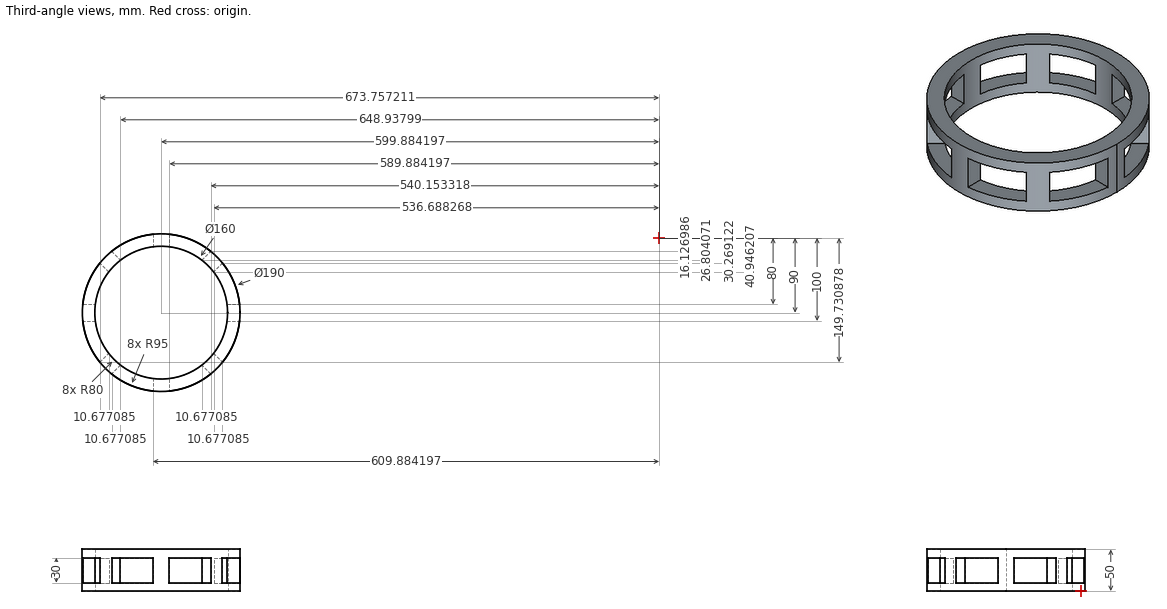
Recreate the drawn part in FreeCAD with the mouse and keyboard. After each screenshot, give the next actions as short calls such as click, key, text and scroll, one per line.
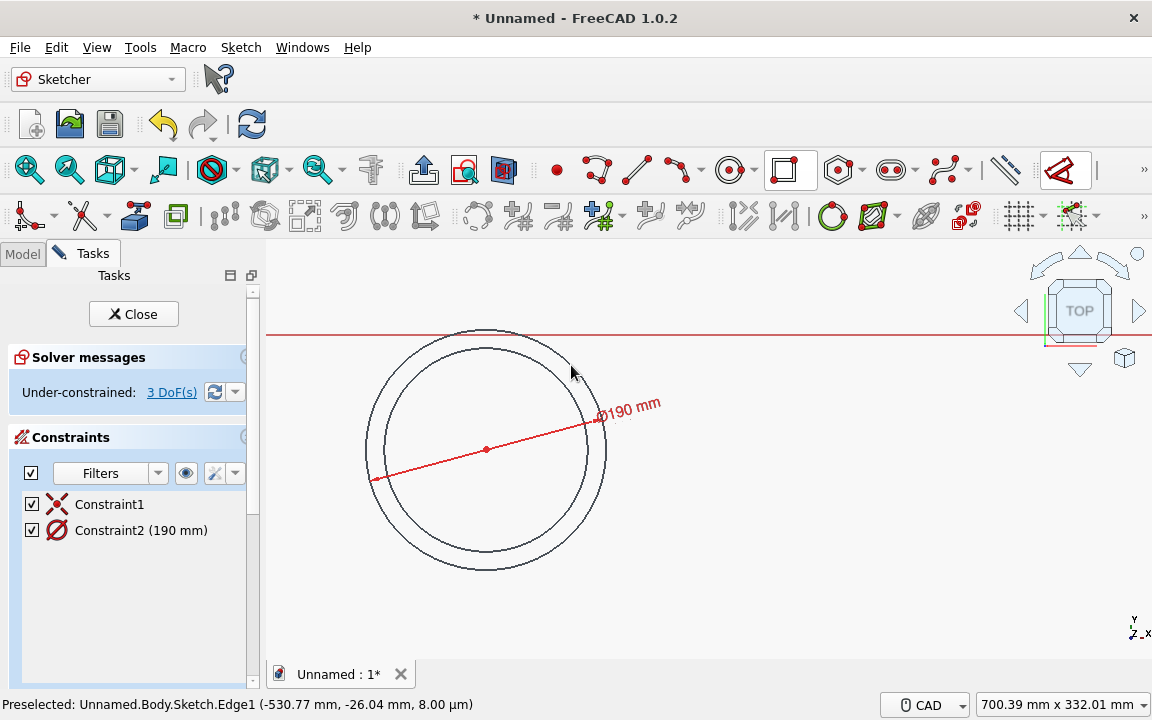
click(558, 378)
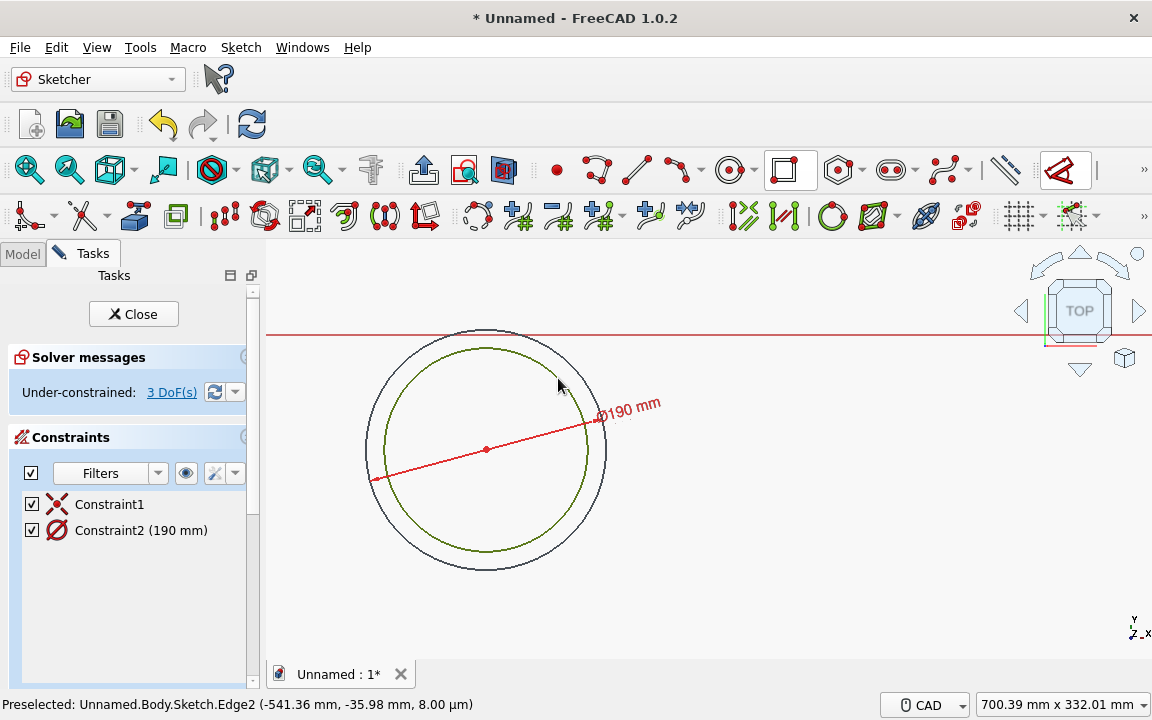
key(k)
key(o)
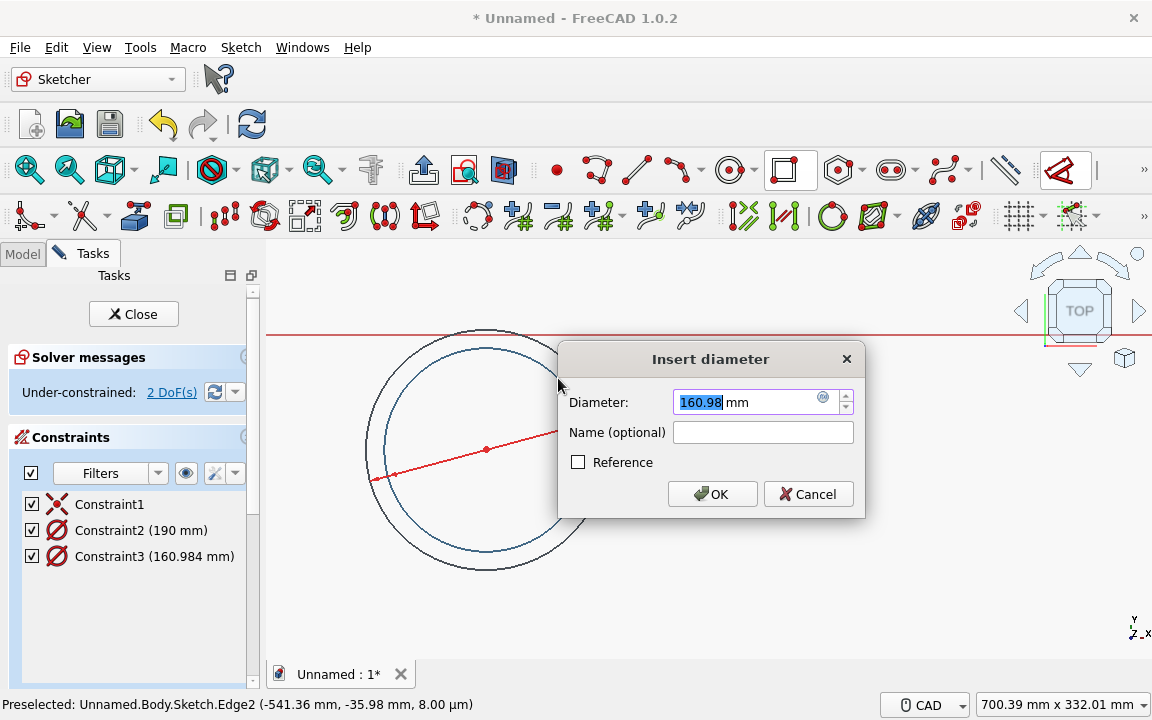
text(160)
key(Return)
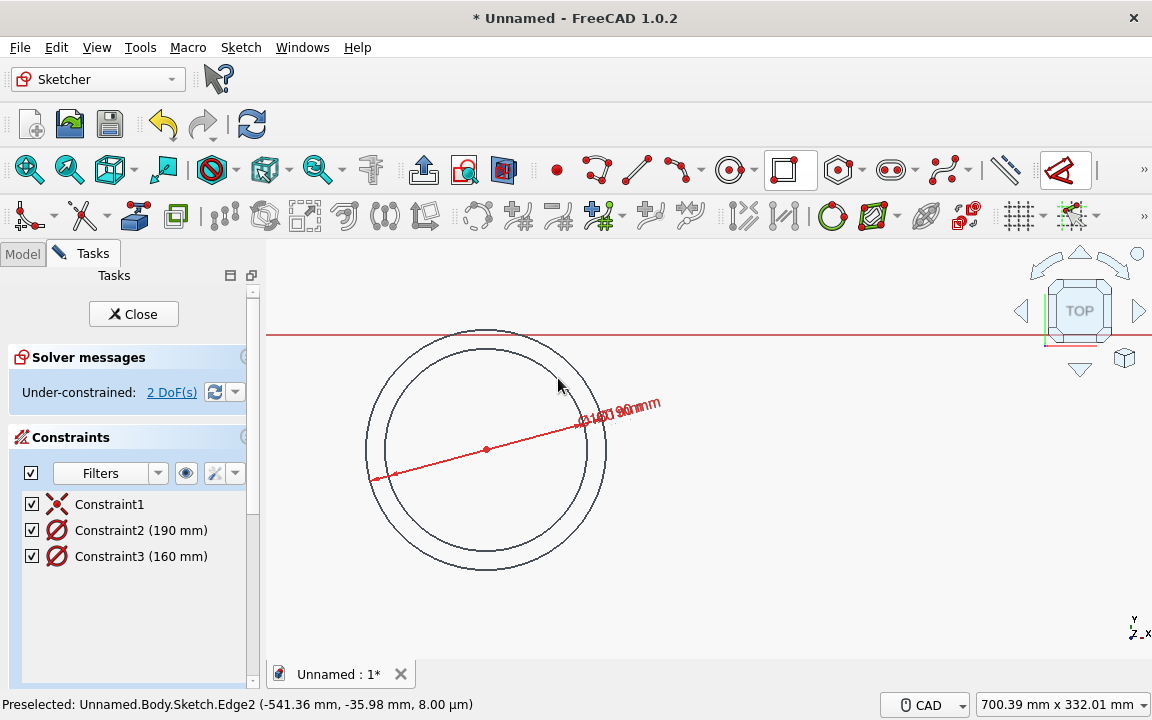
click(486, 450)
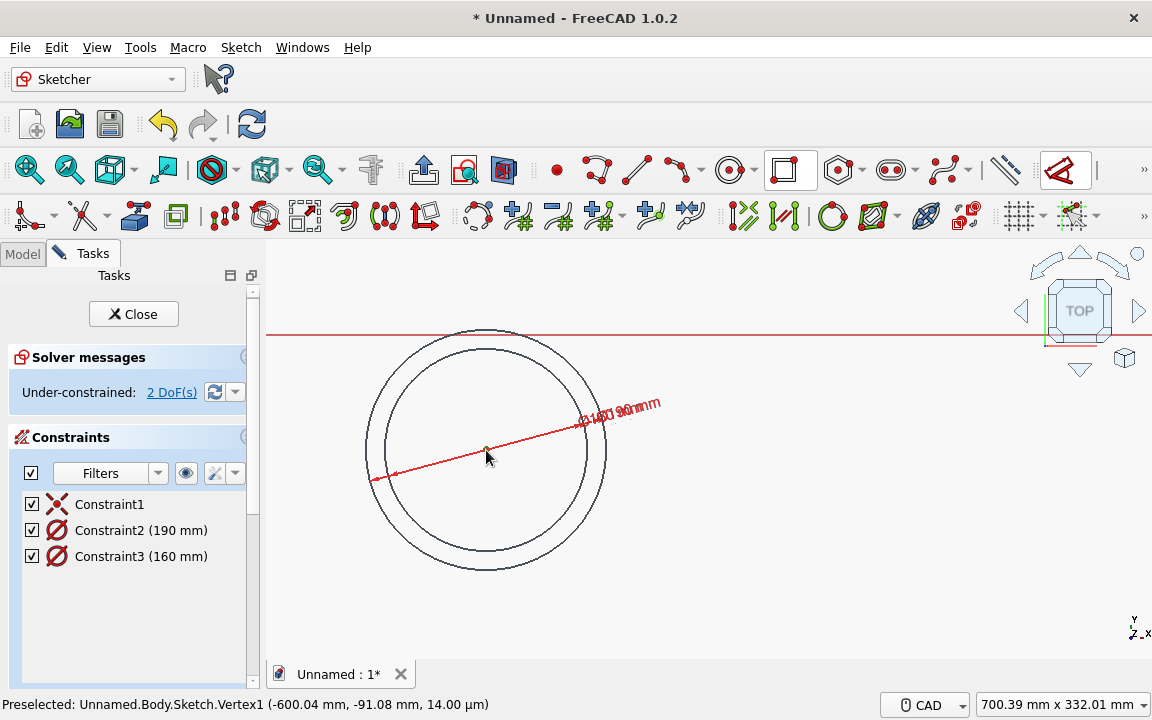
key(i)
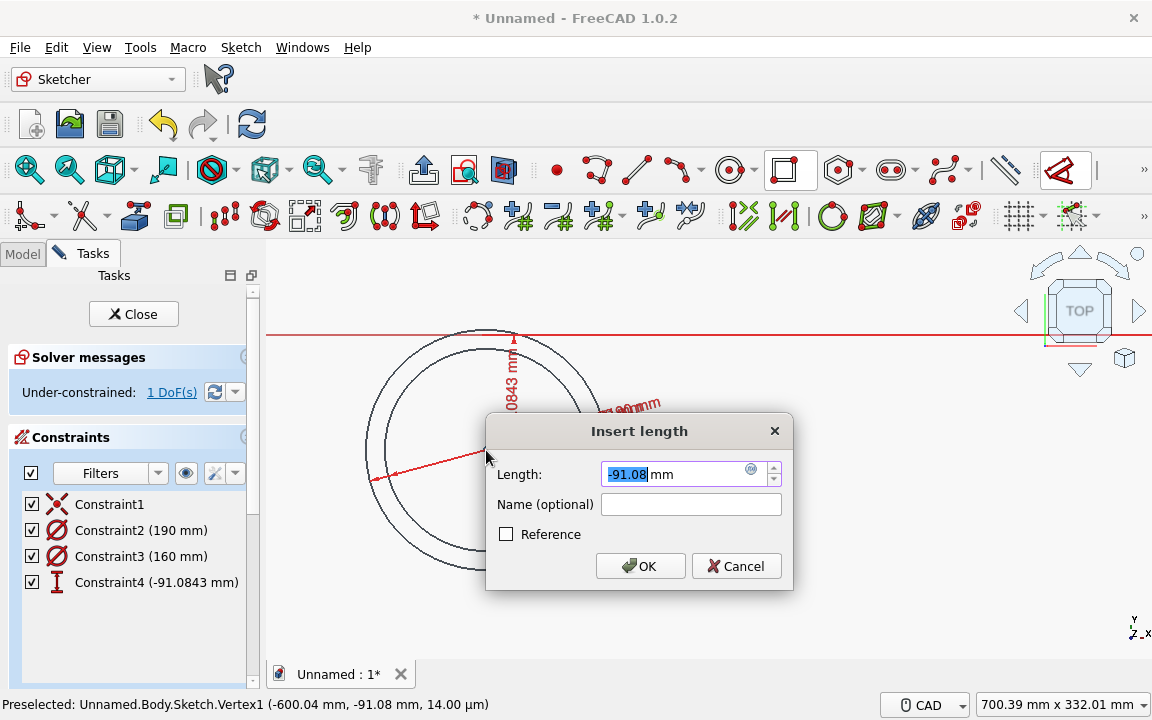
text(-90)
key(Return)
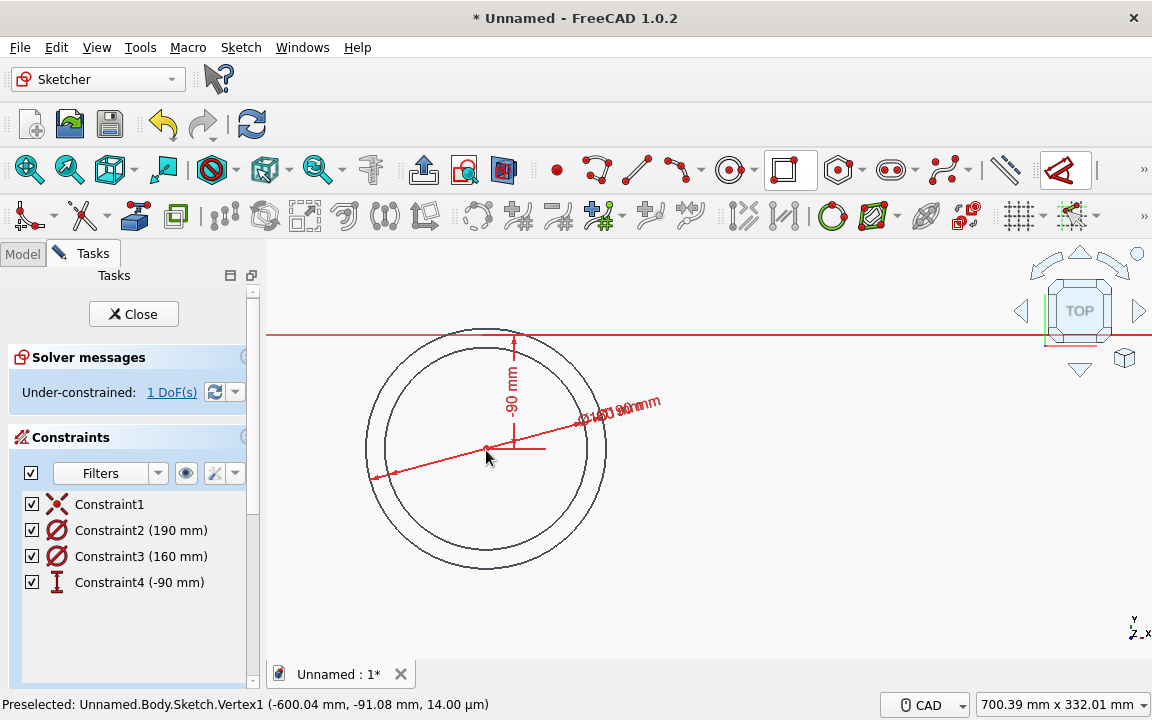
click(486, 449)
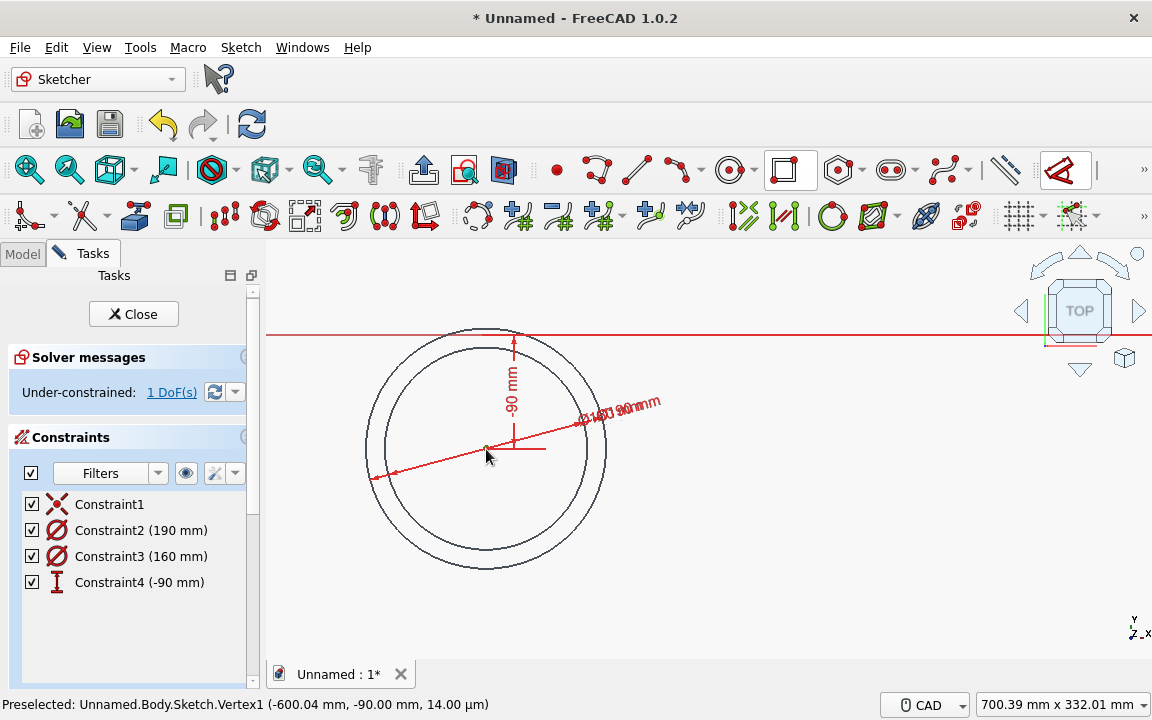
key(l)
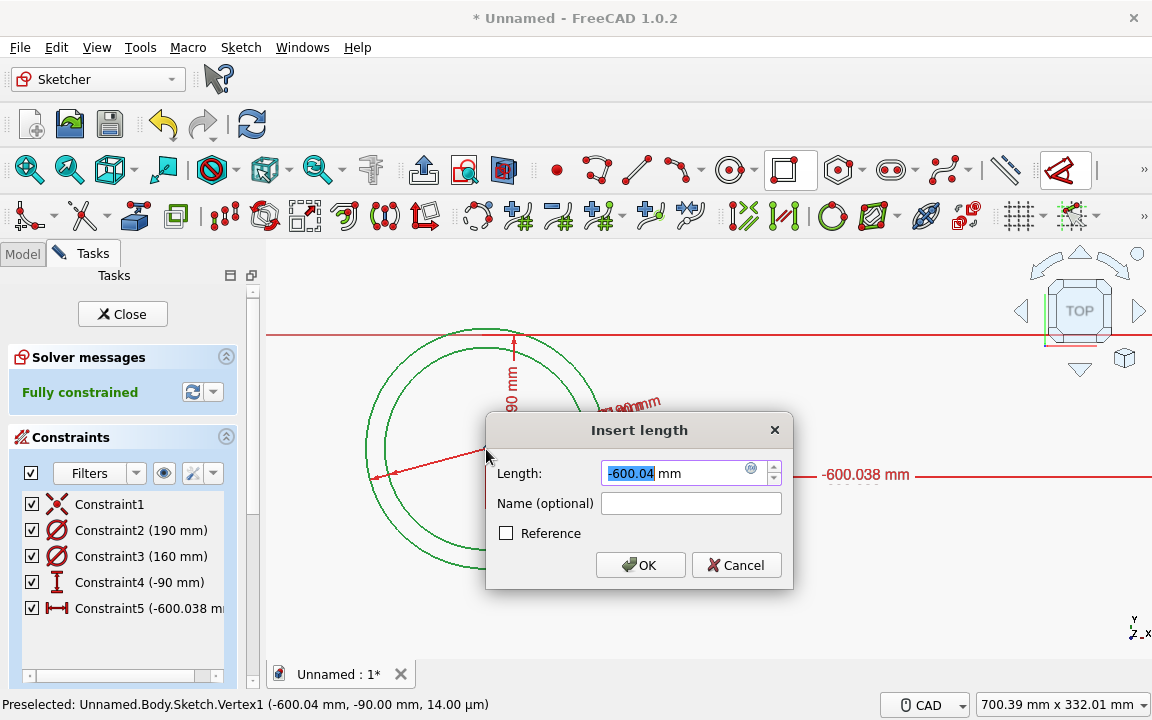
text(-599.884197)
key(Return)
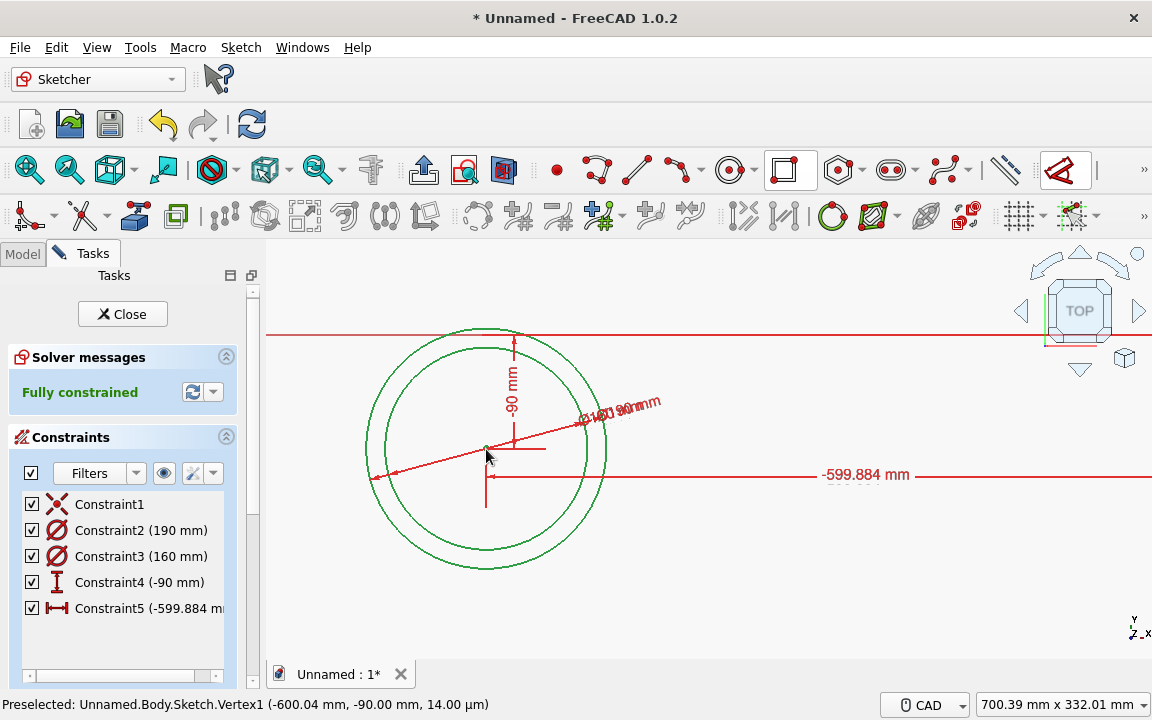
click(123, 314)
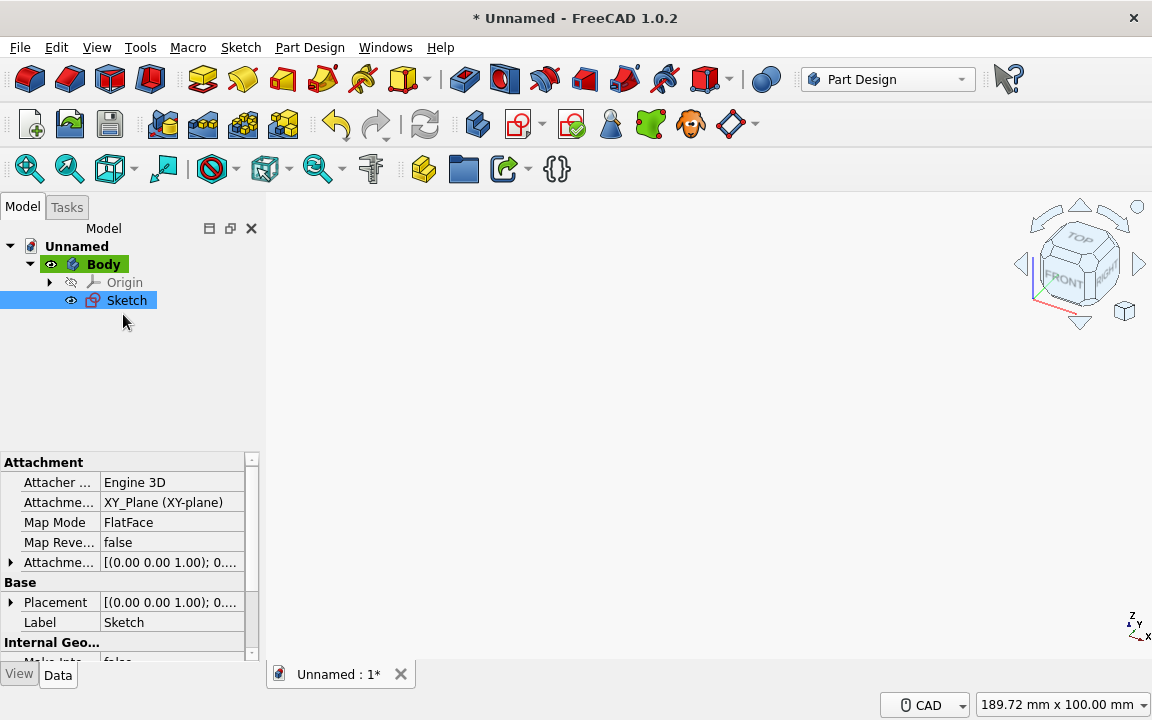
click(204, 80)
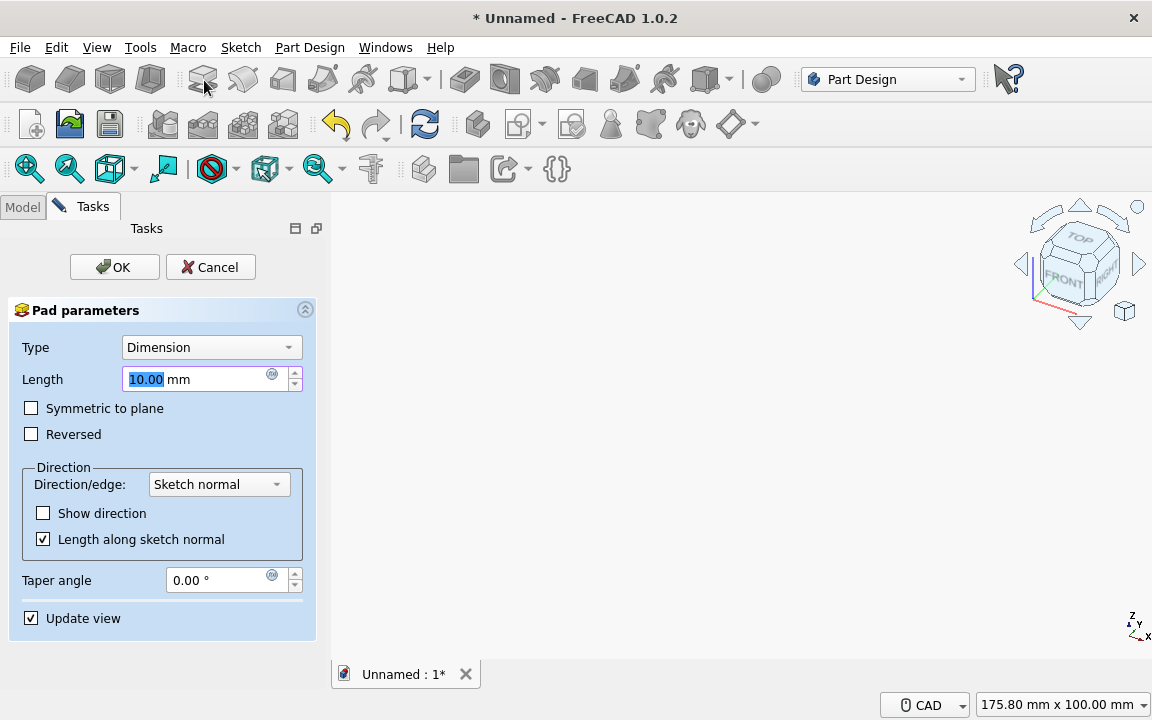
text(50)
key(Tab)